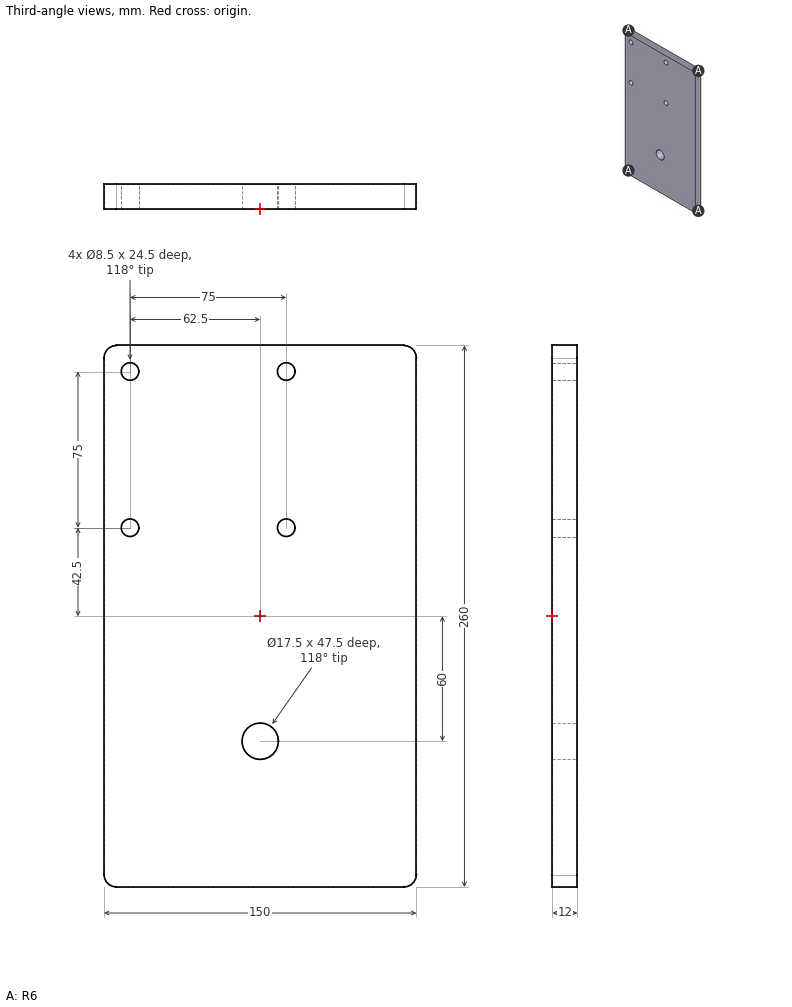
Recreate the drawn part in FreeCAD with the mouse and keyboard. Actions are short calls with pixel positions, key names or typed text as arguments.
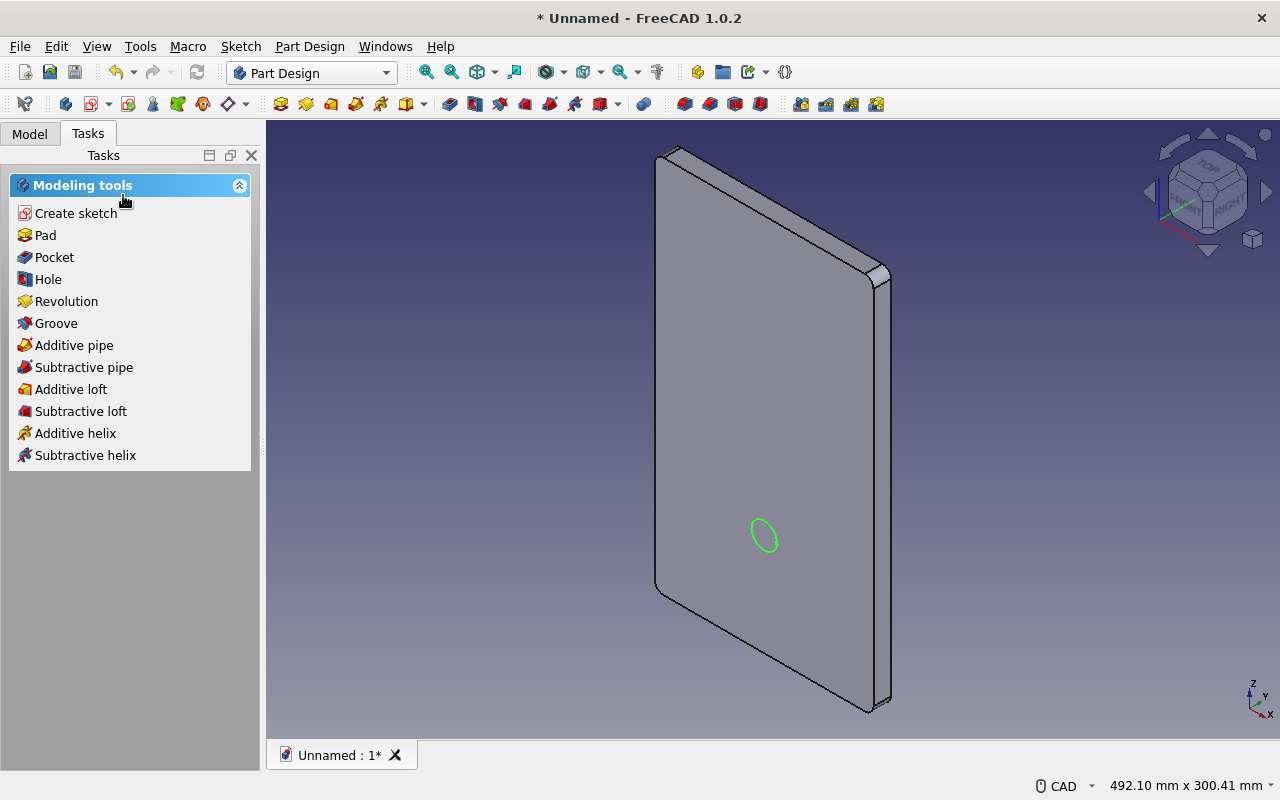
click(475, 104)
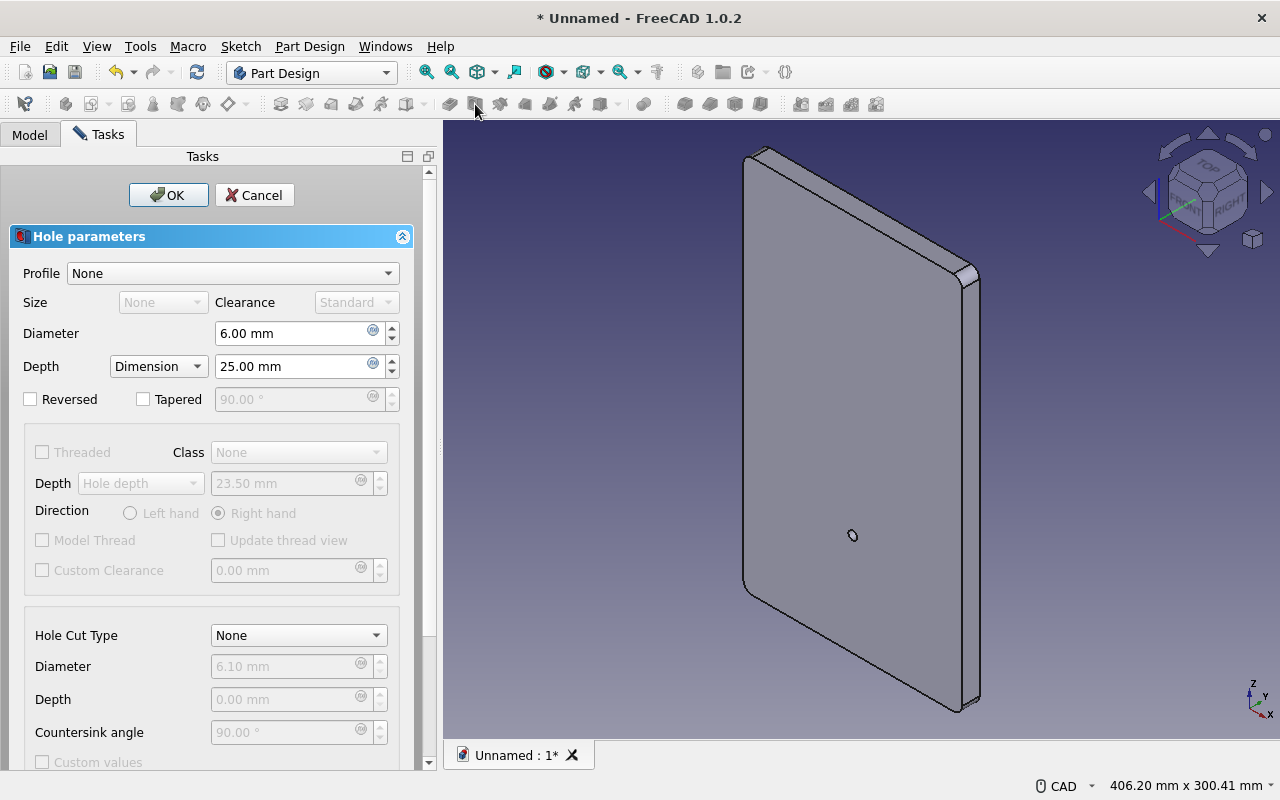
triple_click(300, 334)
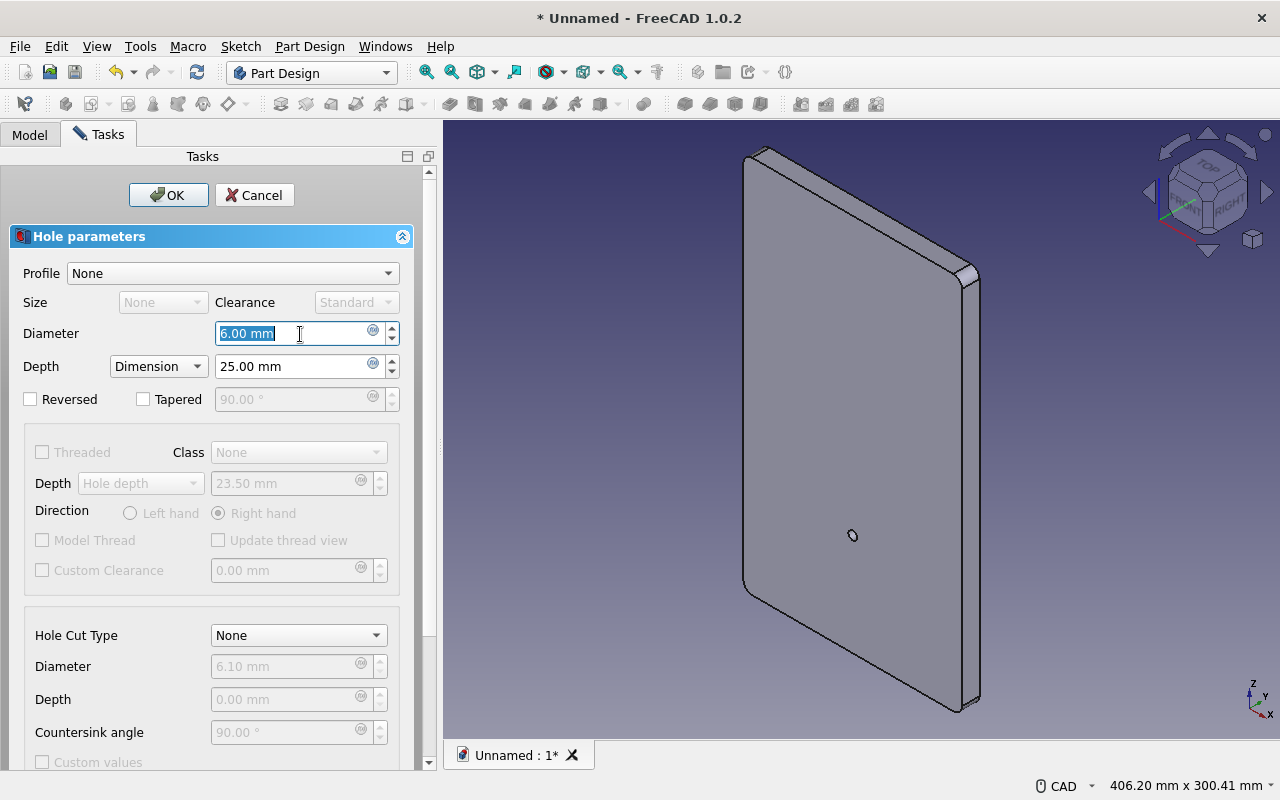
text(17.5)
key(Tab)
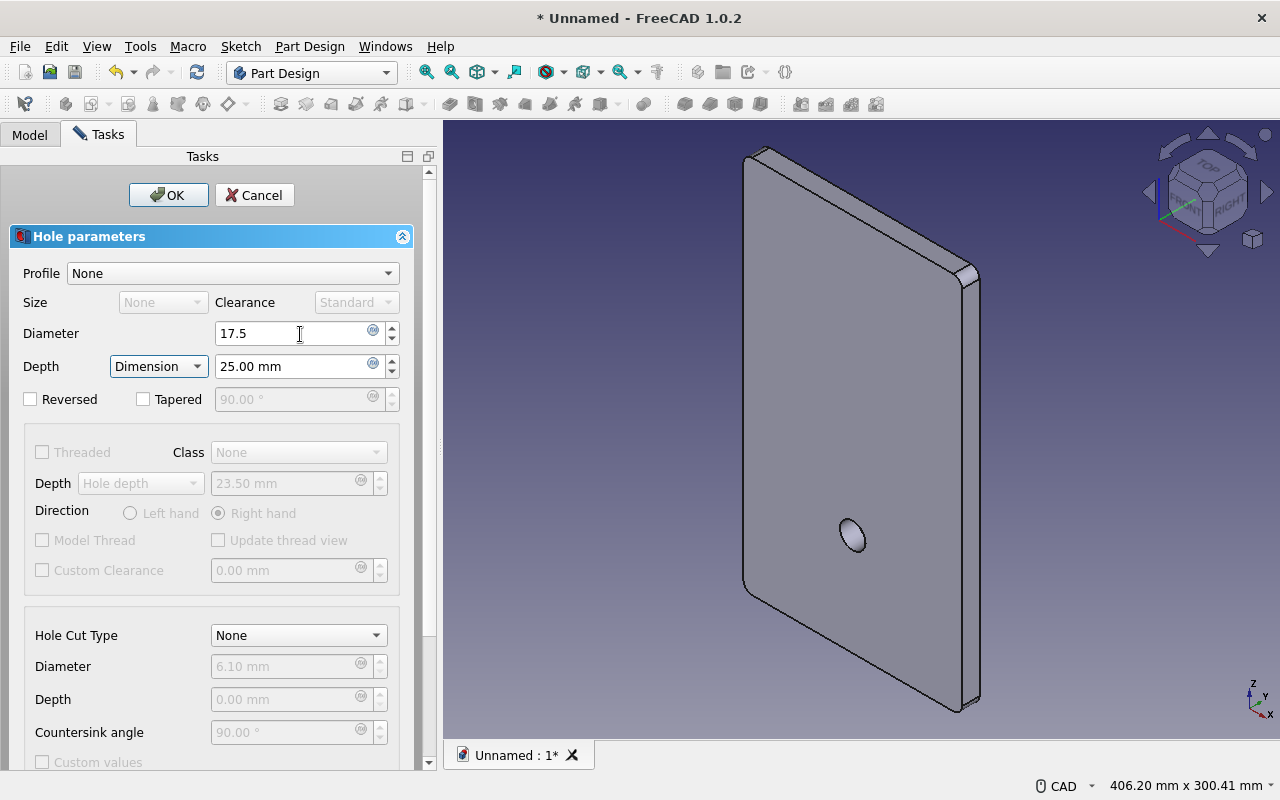
triple_click(300, 366)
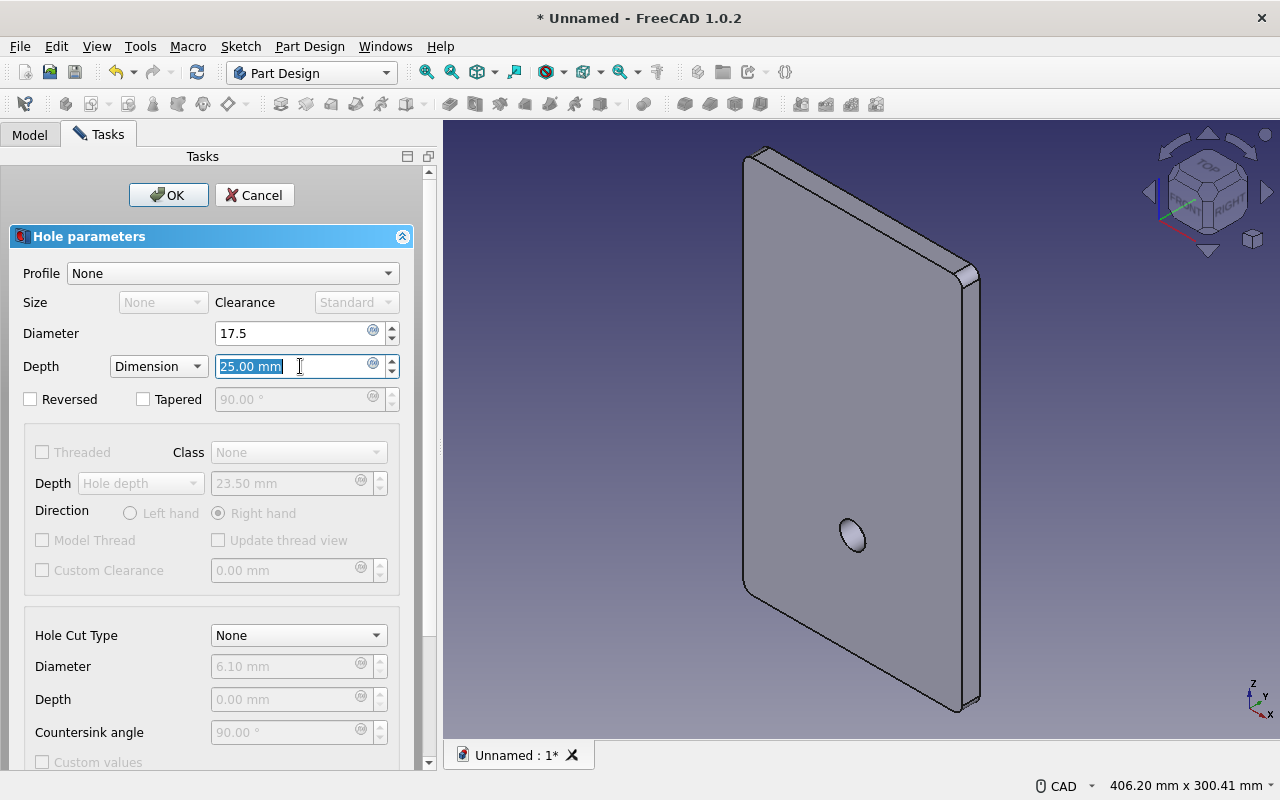
text(47.5)
key(Tab)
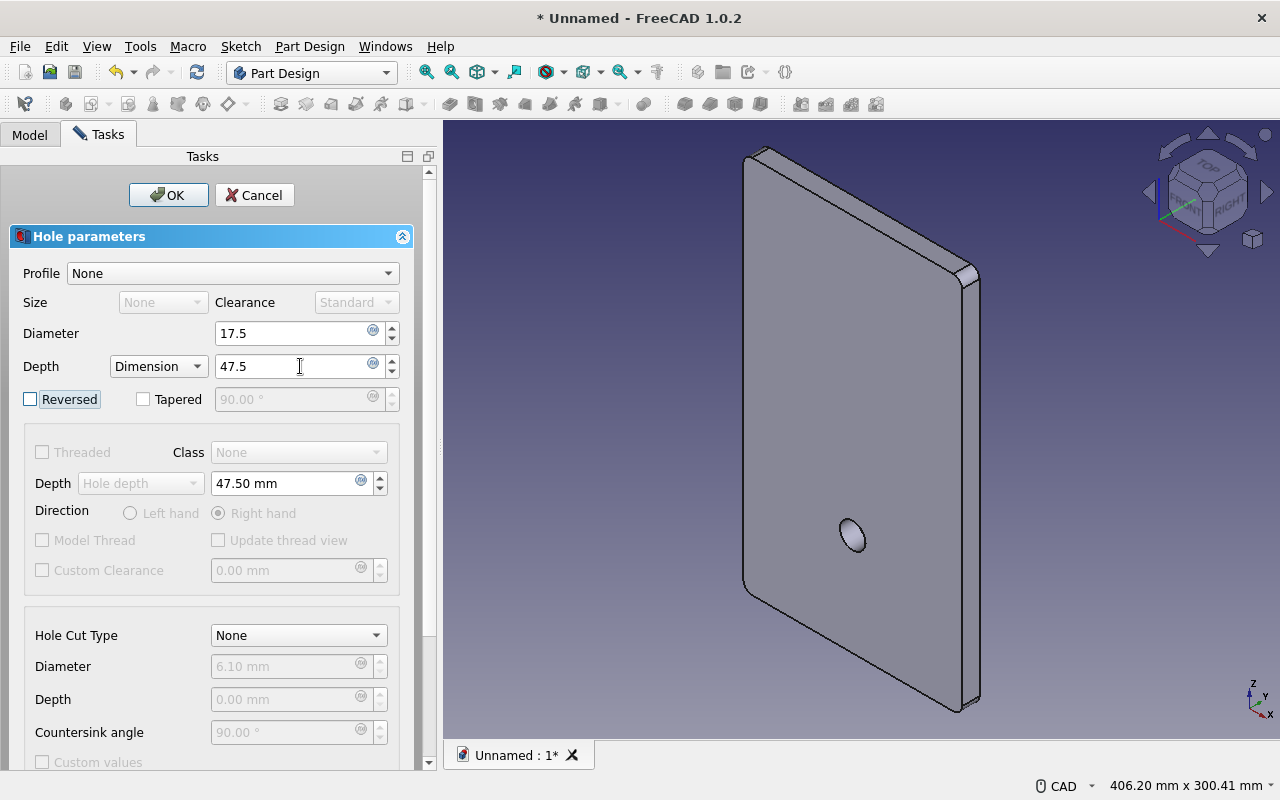
click(169, 195)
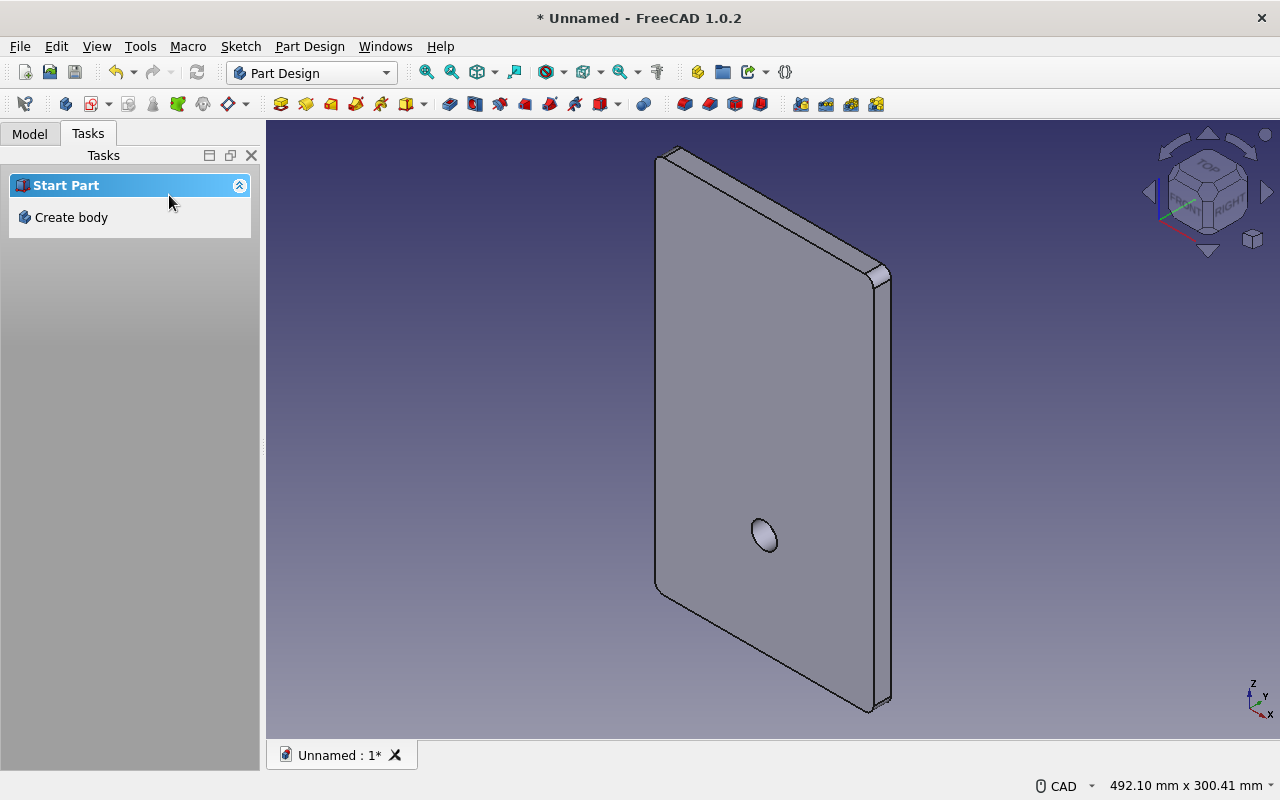
click(764, 371)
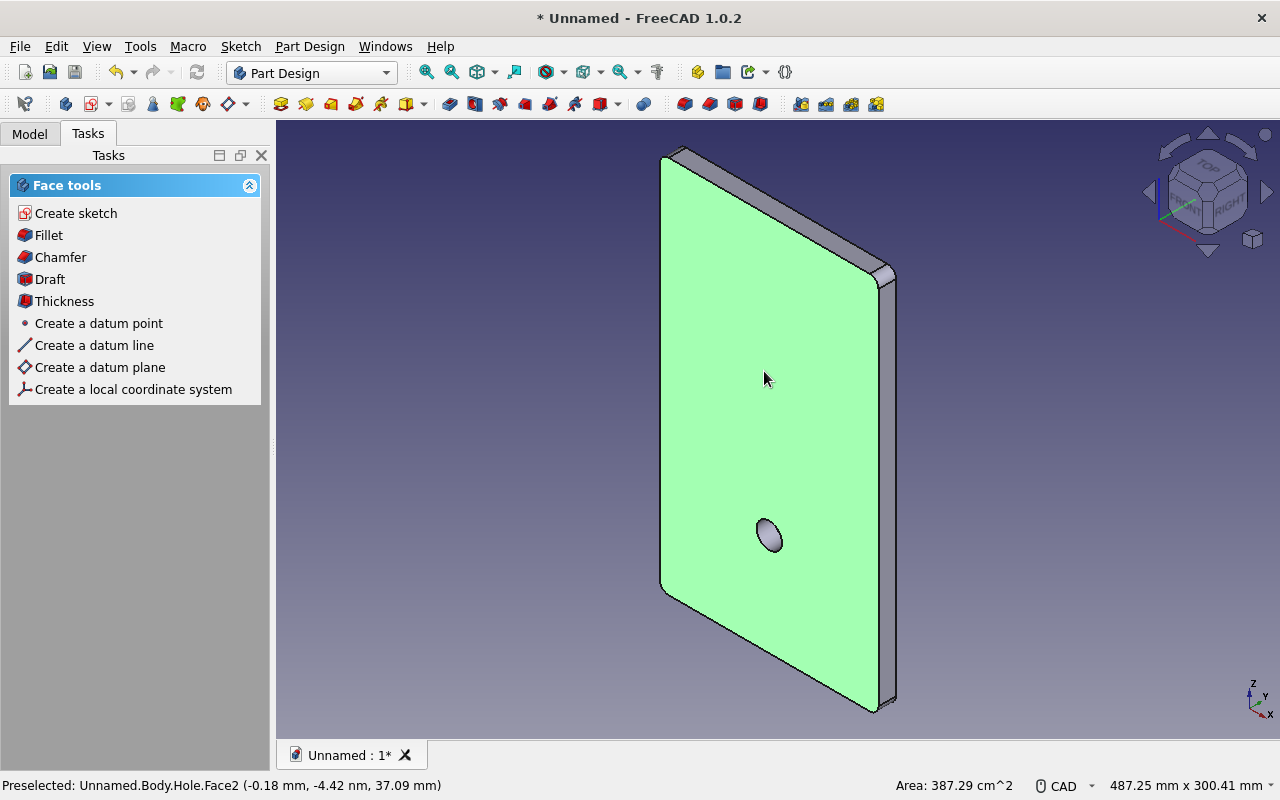
click(90, 104)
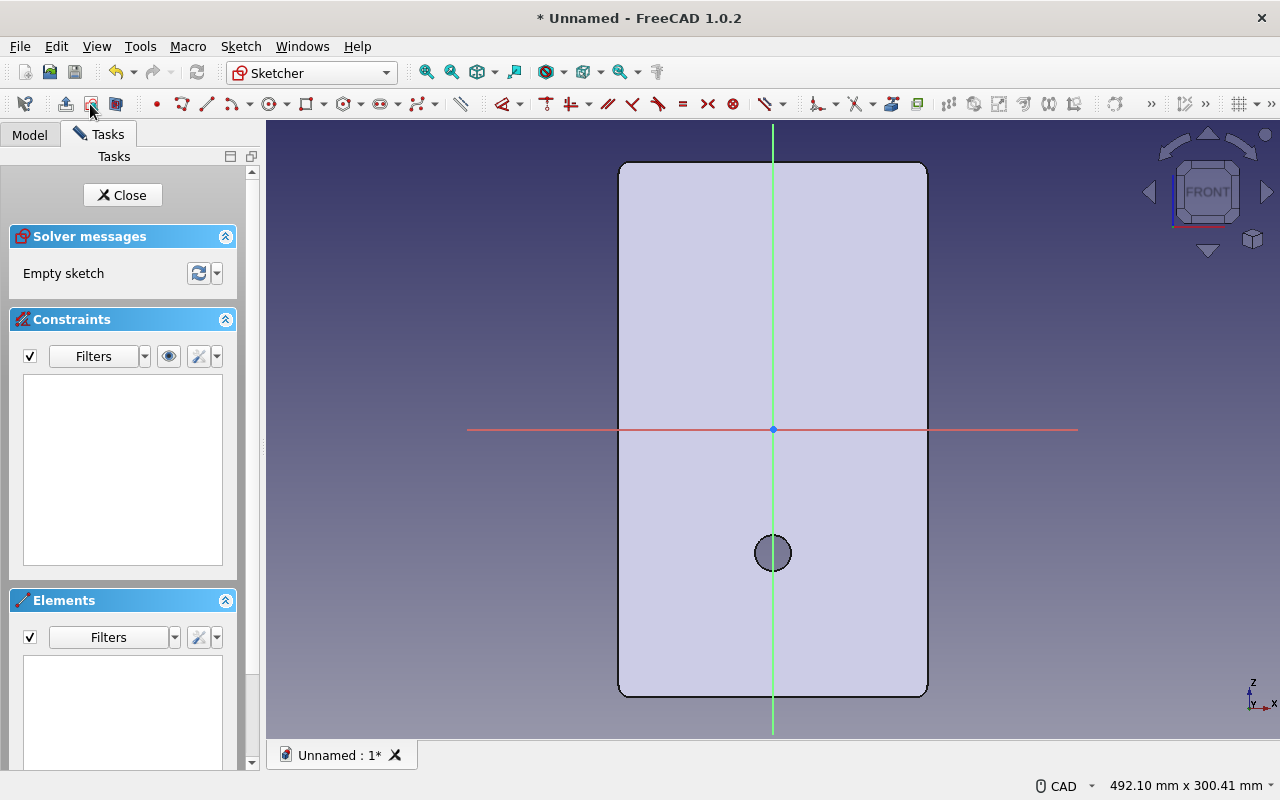
scroll(756, 148, up, 2)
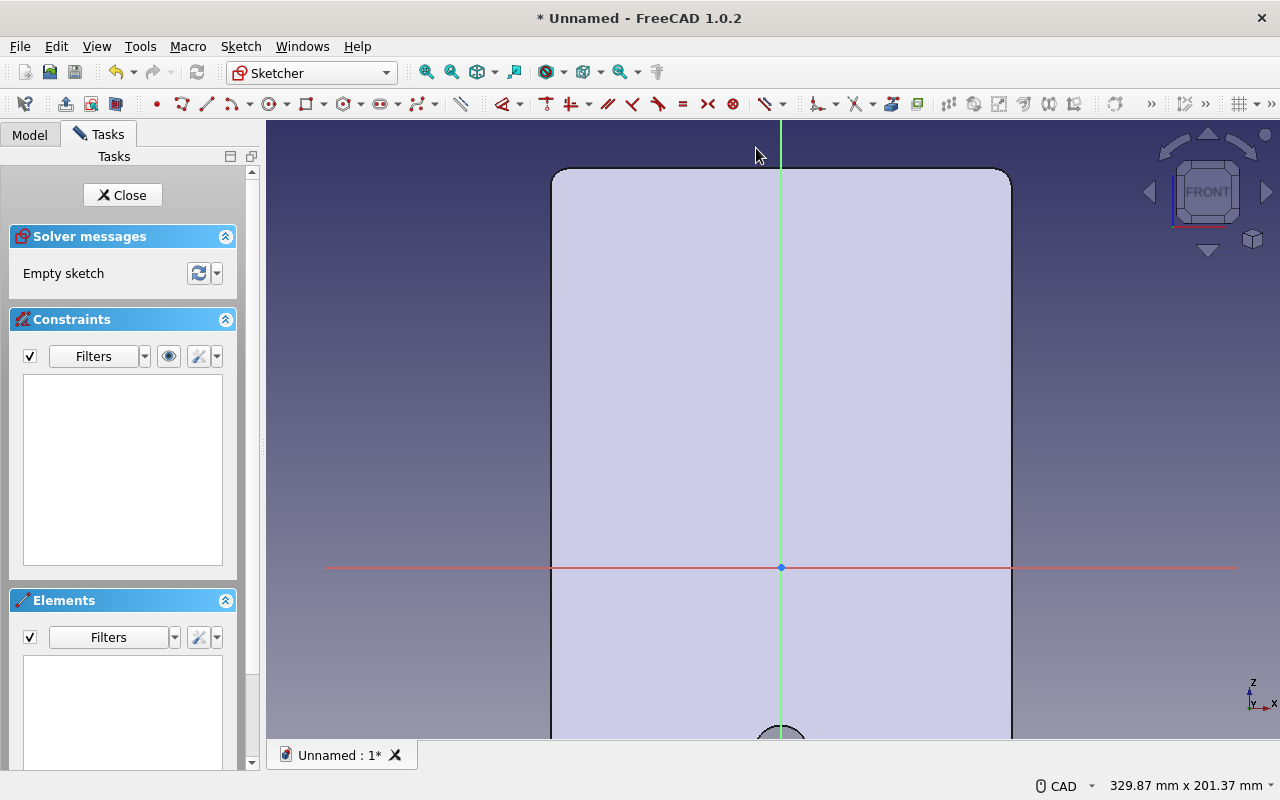
click(268, 104)